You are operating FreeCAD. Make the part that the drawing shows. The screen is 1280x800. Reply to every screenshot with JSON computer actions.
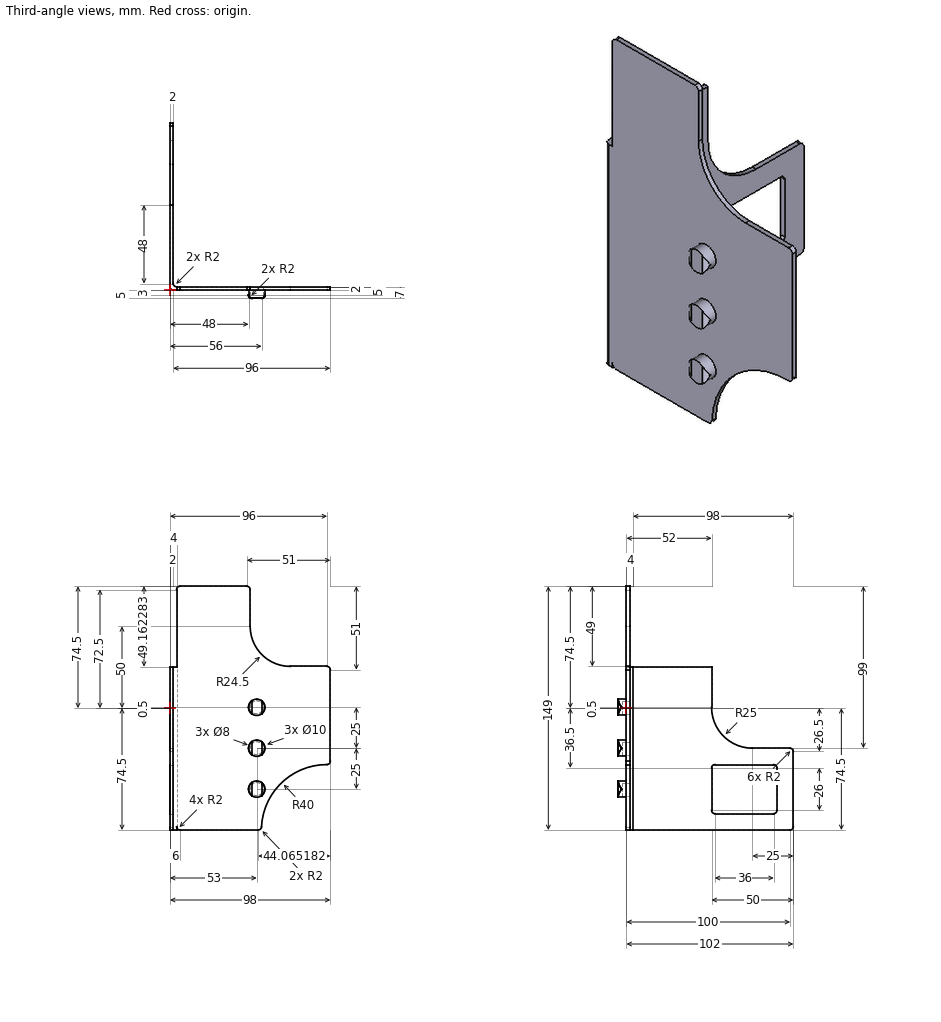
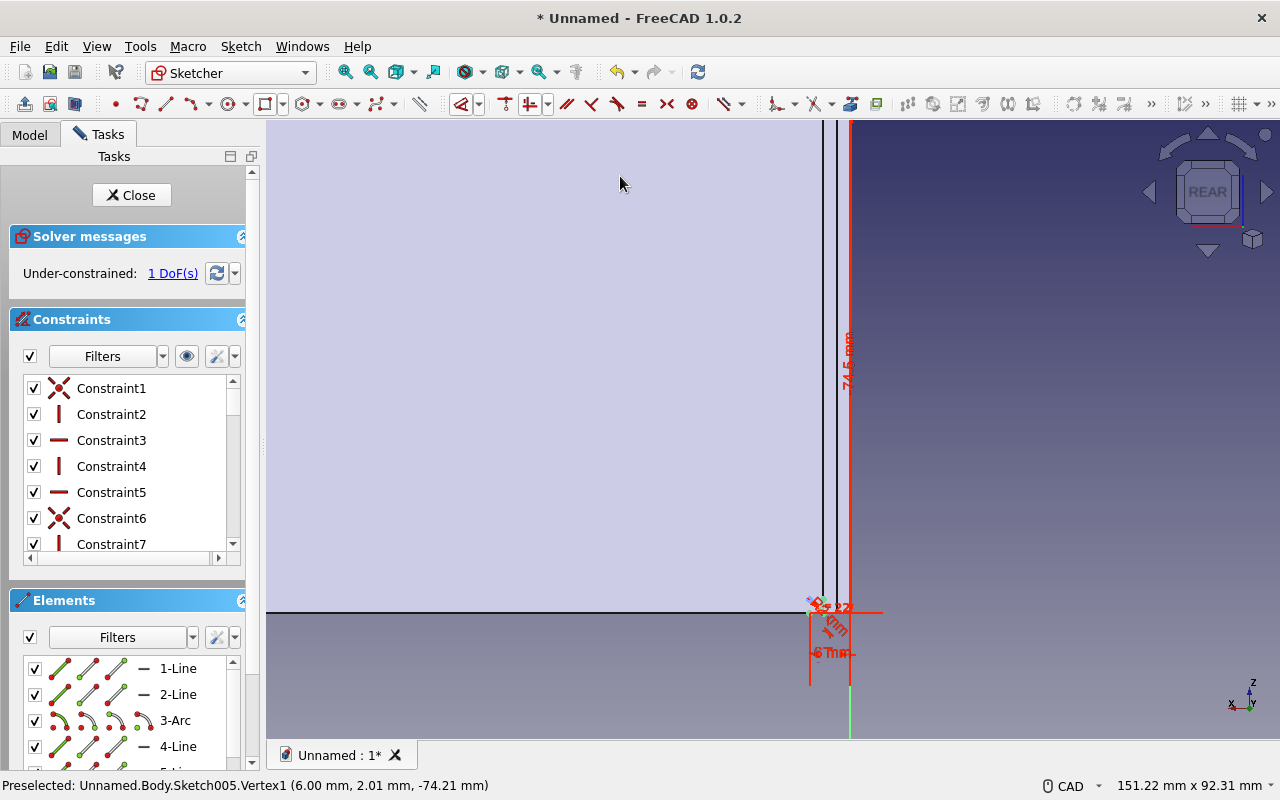
{"action": "scroll", "coordinate": [811, 613], "scroll_direction": "down", "scroll_amount": 5}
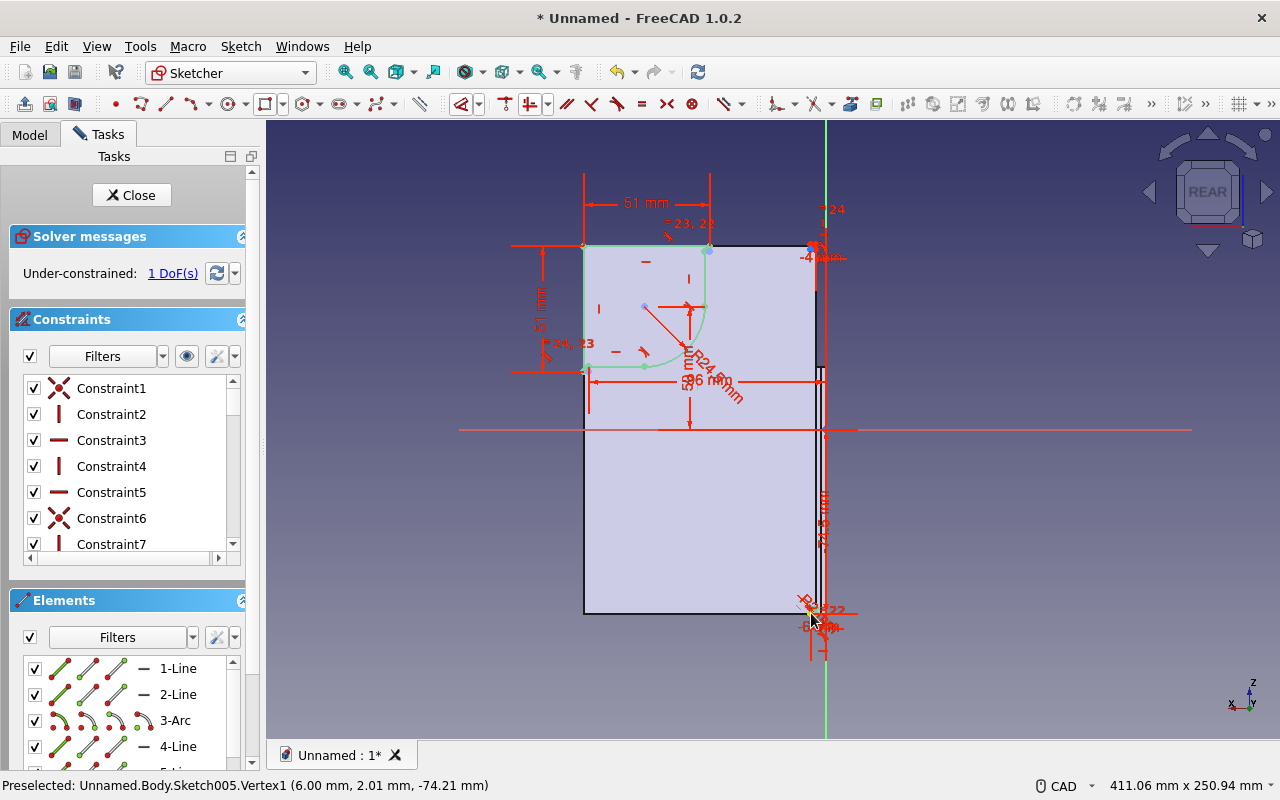
{"action": "scroll", "coordinate": [816, 249], "scroll_direction": "up", "scroll_amount": 5}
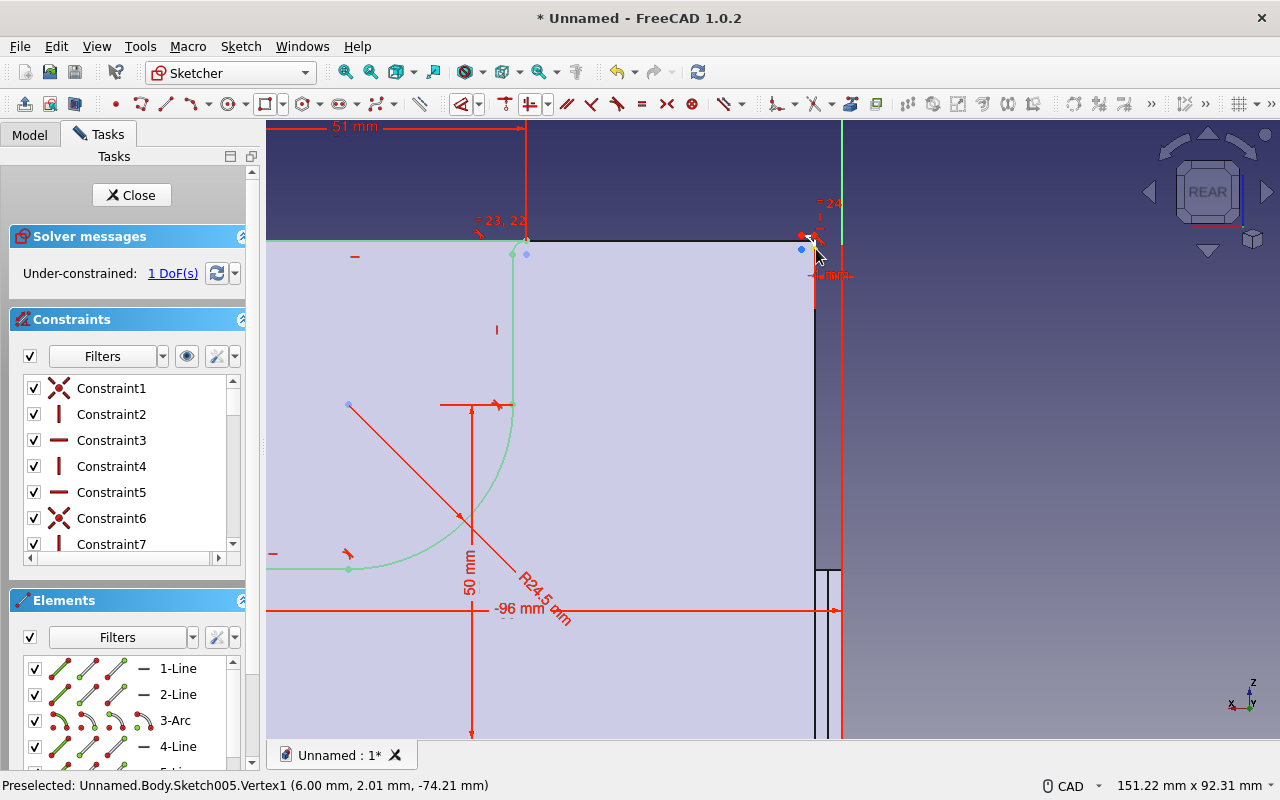
{"action": "left_click", "coordinate": [815, 249]}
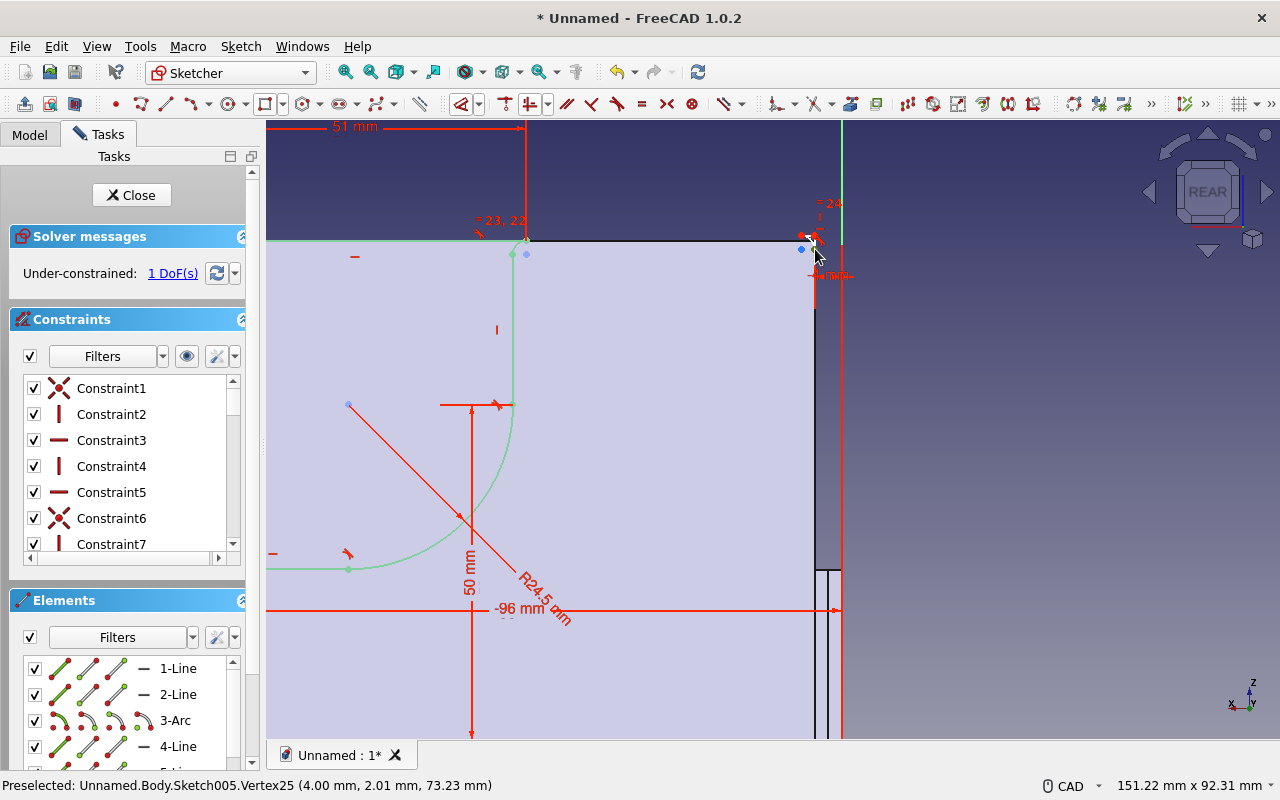
{"action": "key", "text": "i"}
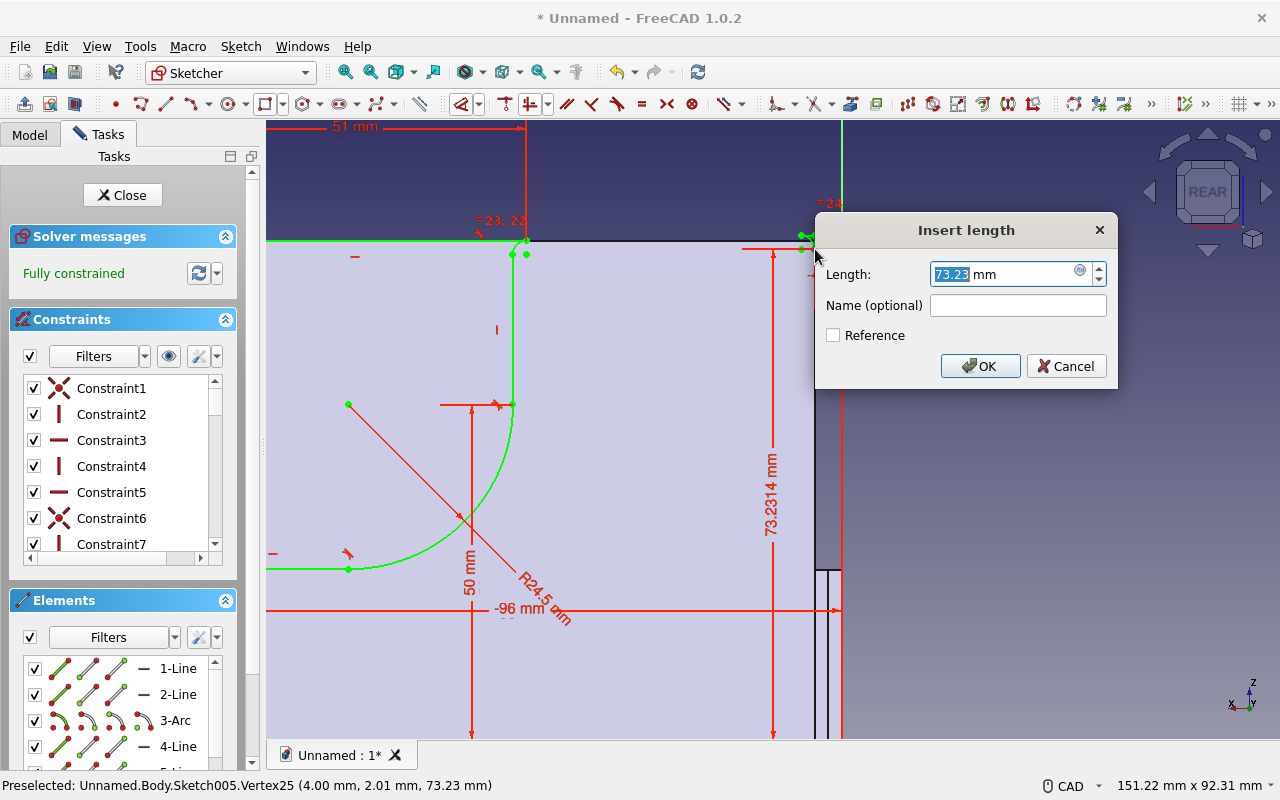
{"action": "type", "text": "72.5"}
{"action": "key", "text": "Return"}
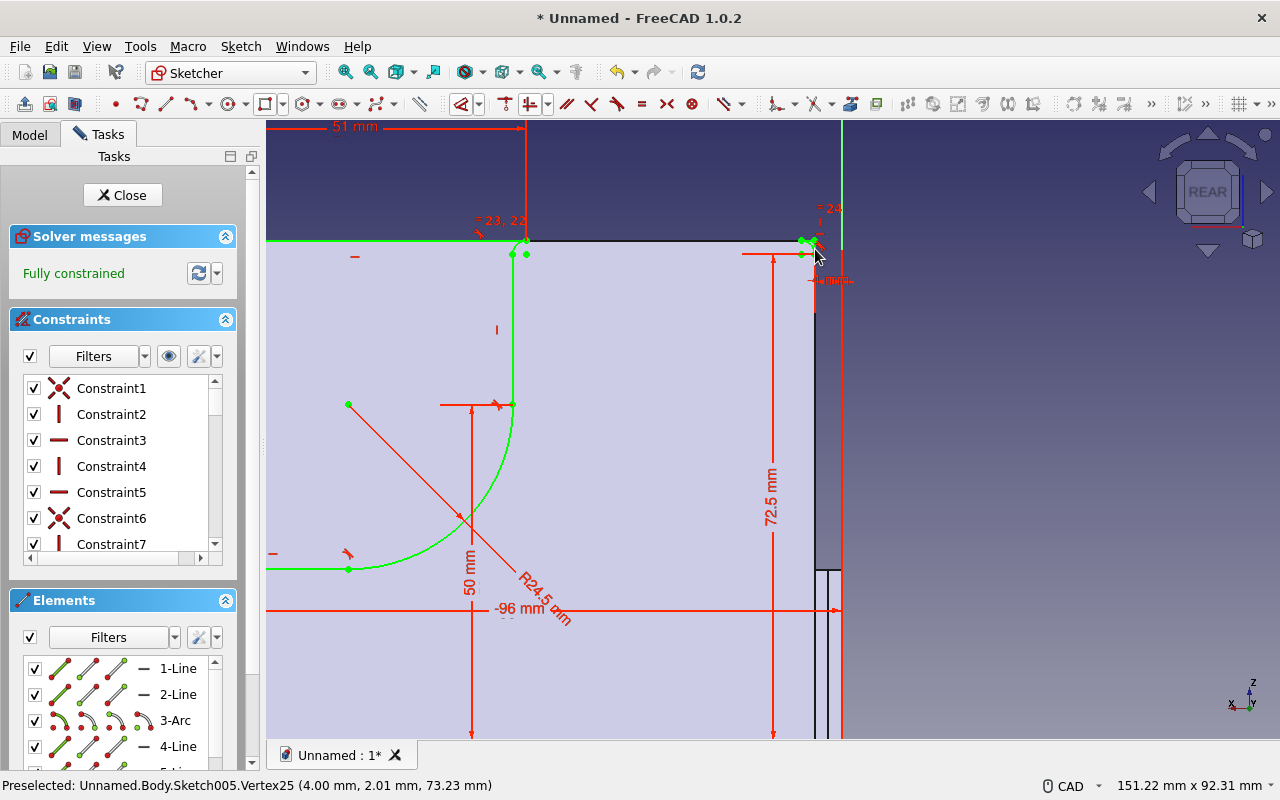
{"action": "left_click", "coordinate": [123, 195]}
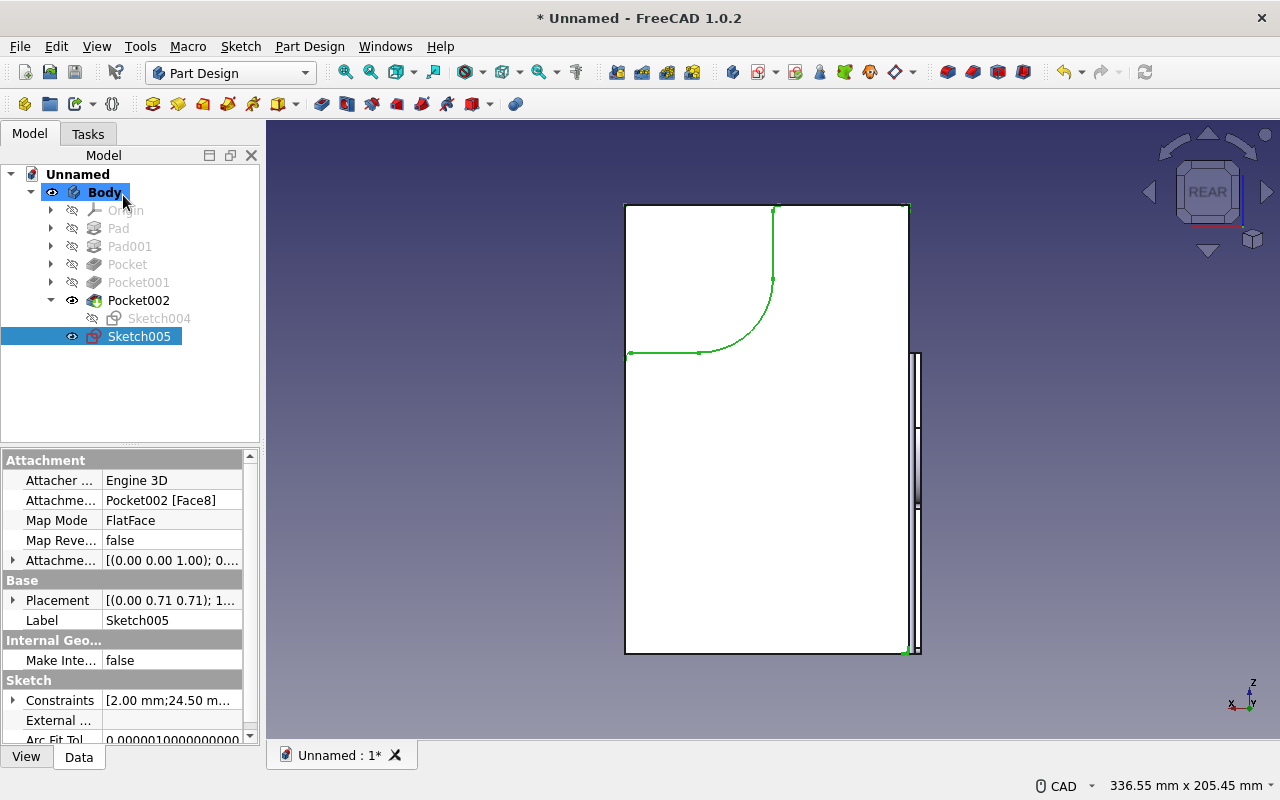
{"action": "left_click", "coordinate": [322, 104]}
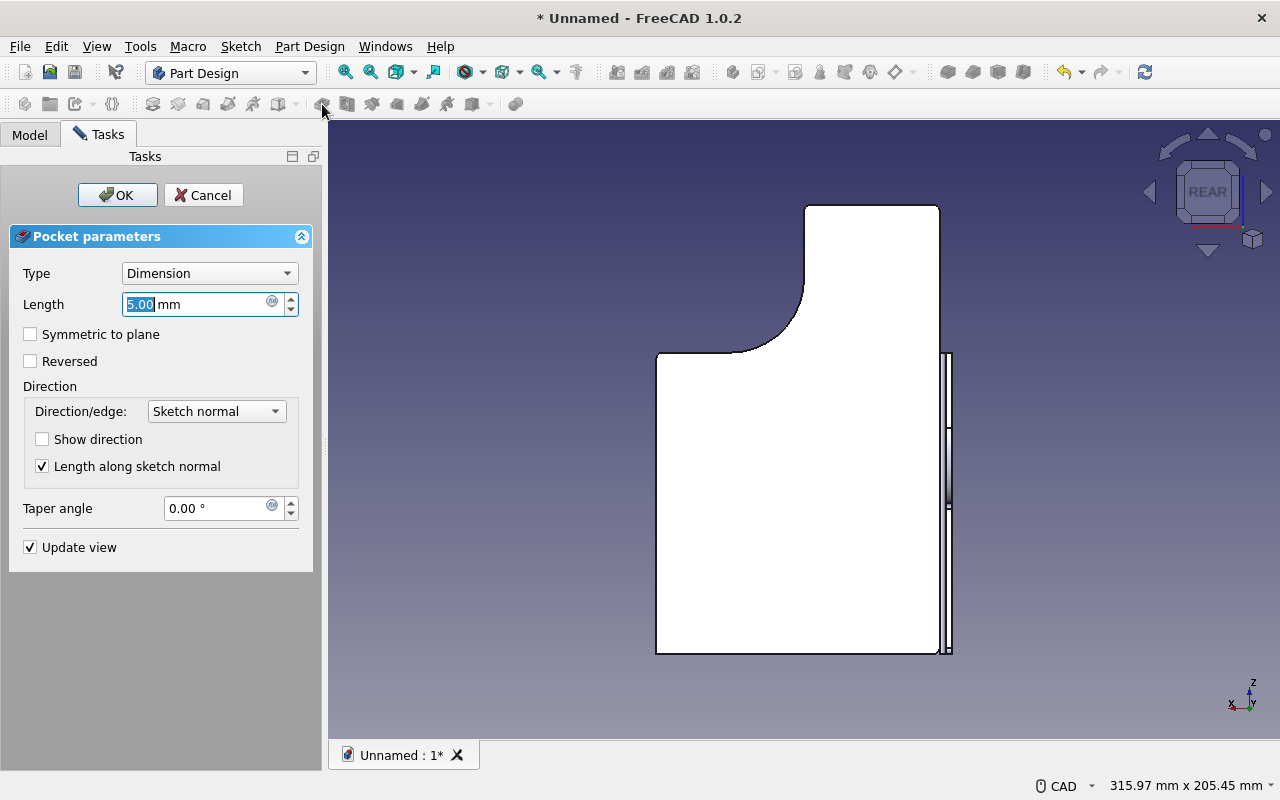
{"action": "type", "text": "2"}
{"action": "key", "text": "Tab"}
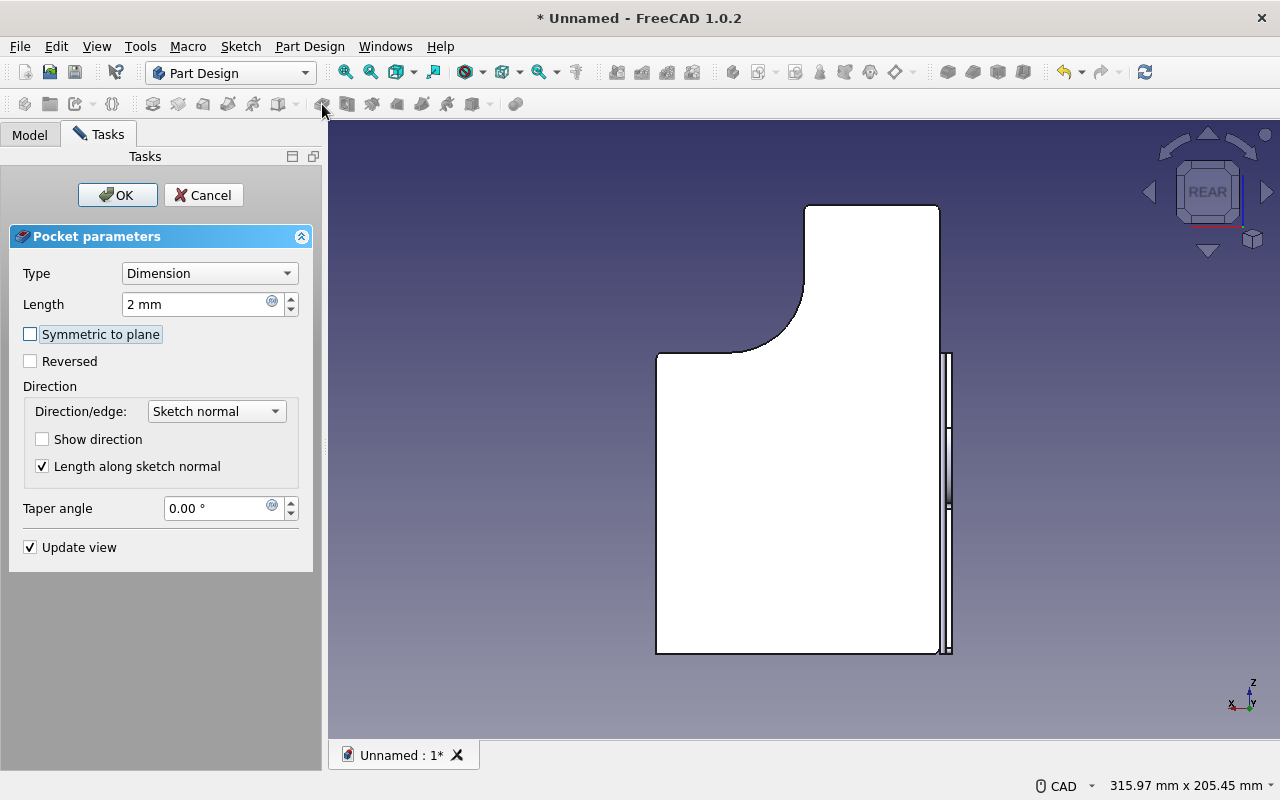
{"action": "left_click", "coordinate": [118, 195]}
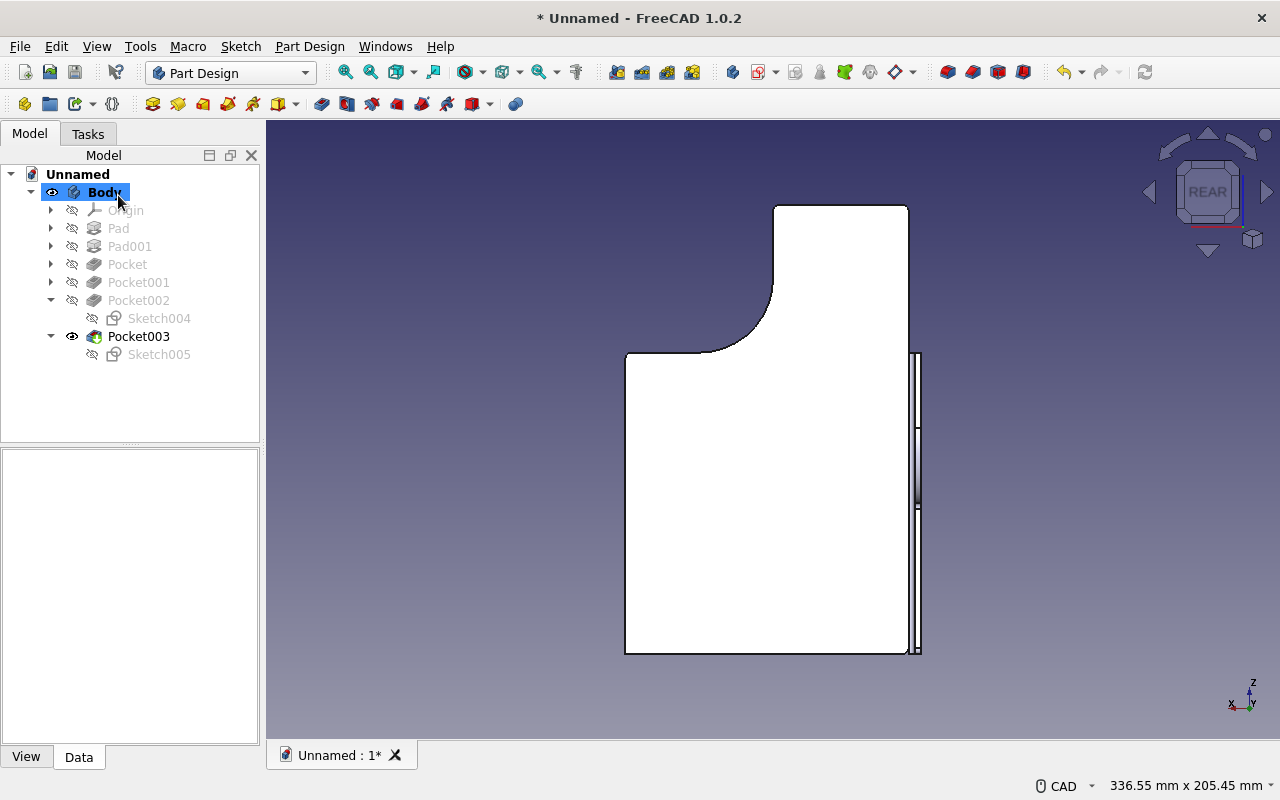
{"action": "left_click", "coordinate": [767, 493]}